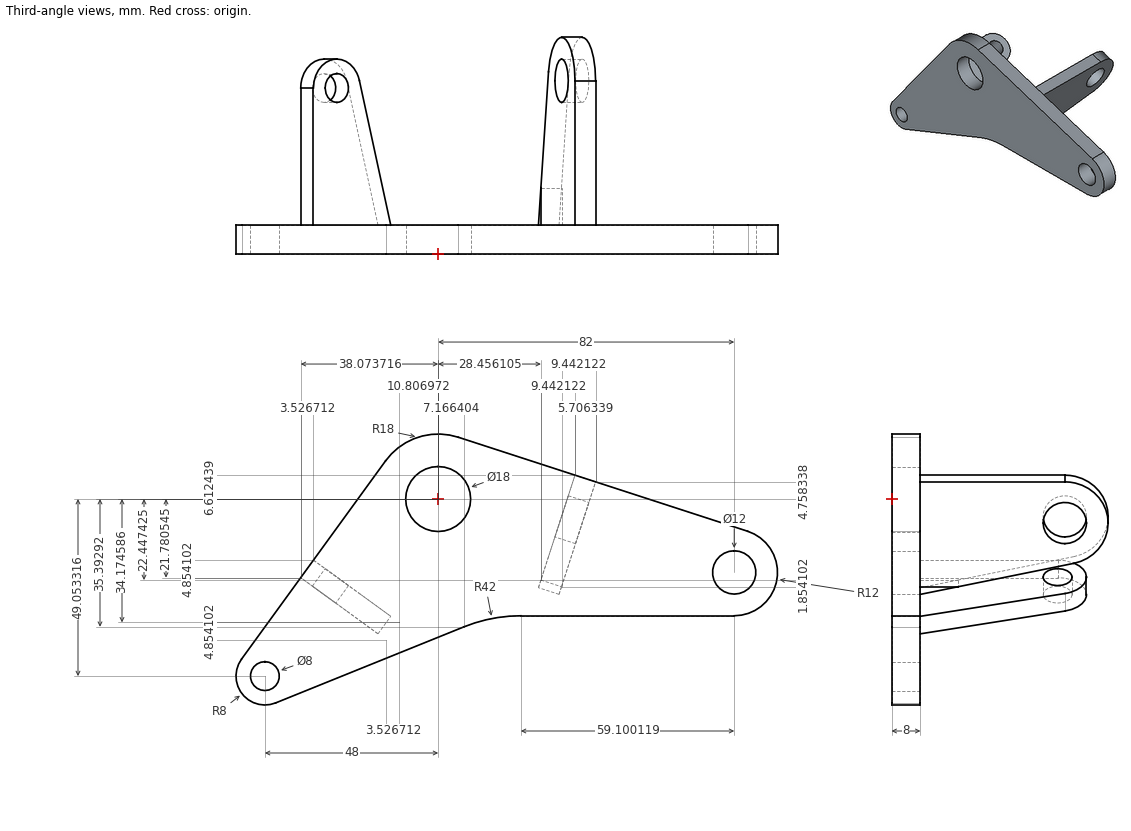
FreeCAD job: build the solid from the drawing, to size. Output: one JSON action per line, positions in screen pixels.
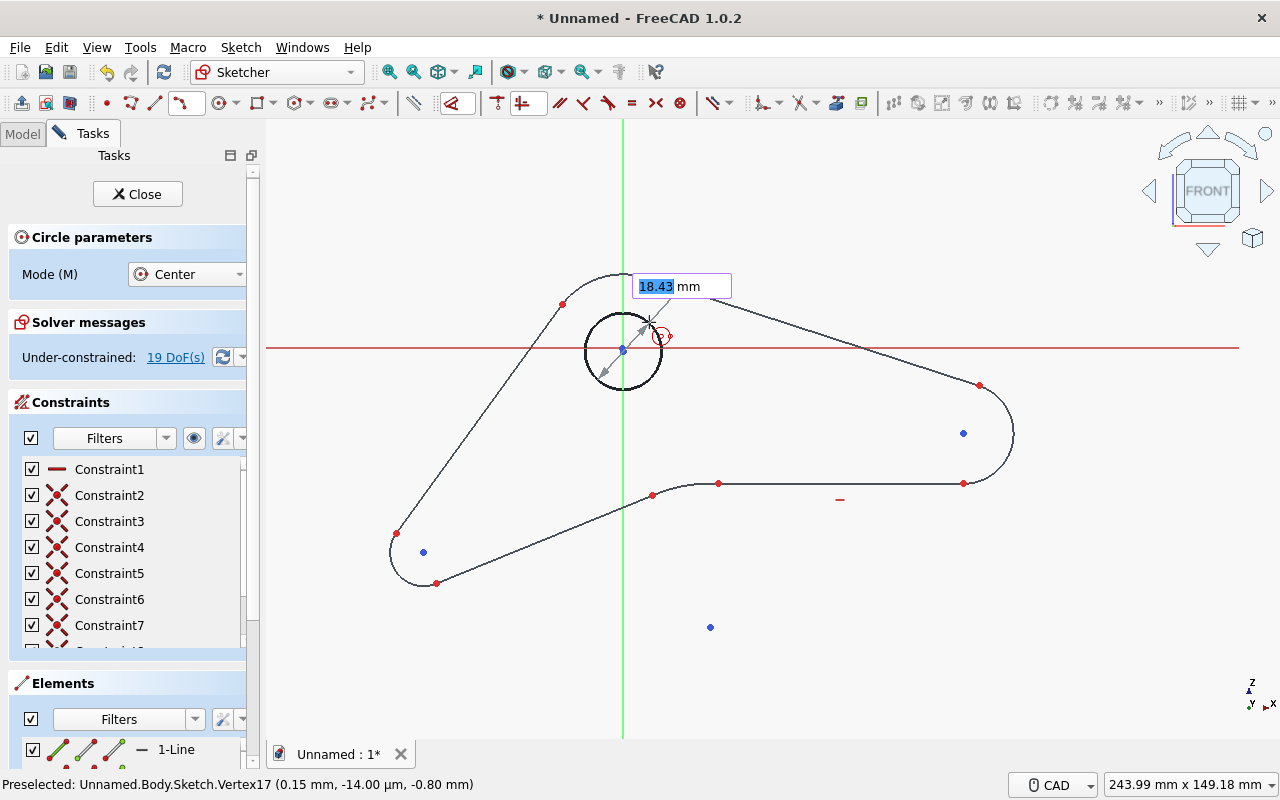
{"action": "type", "text": "18"}
{"action": "key", "text": "Return"}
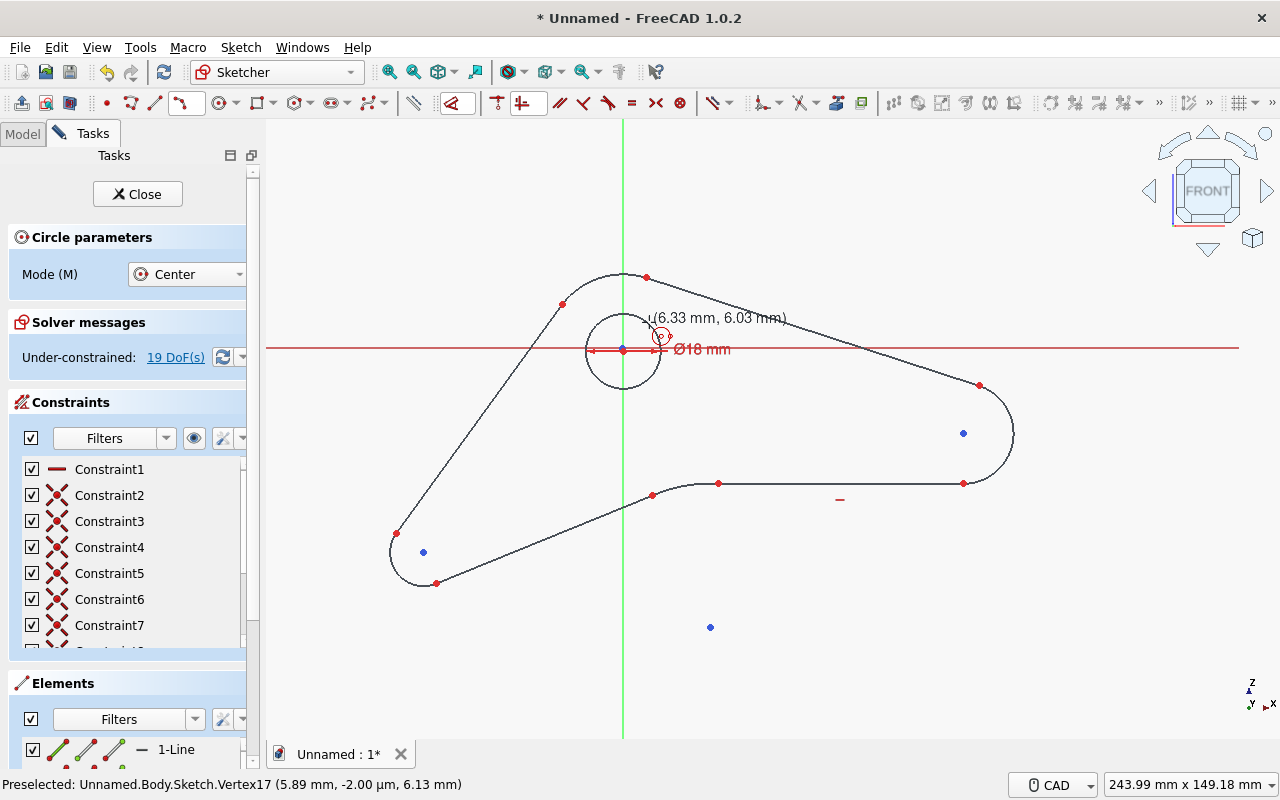
{"action": "left_click", "coordinate": [963, 433]}
{"action": "mouse_move", "coordinate": [981, 415]}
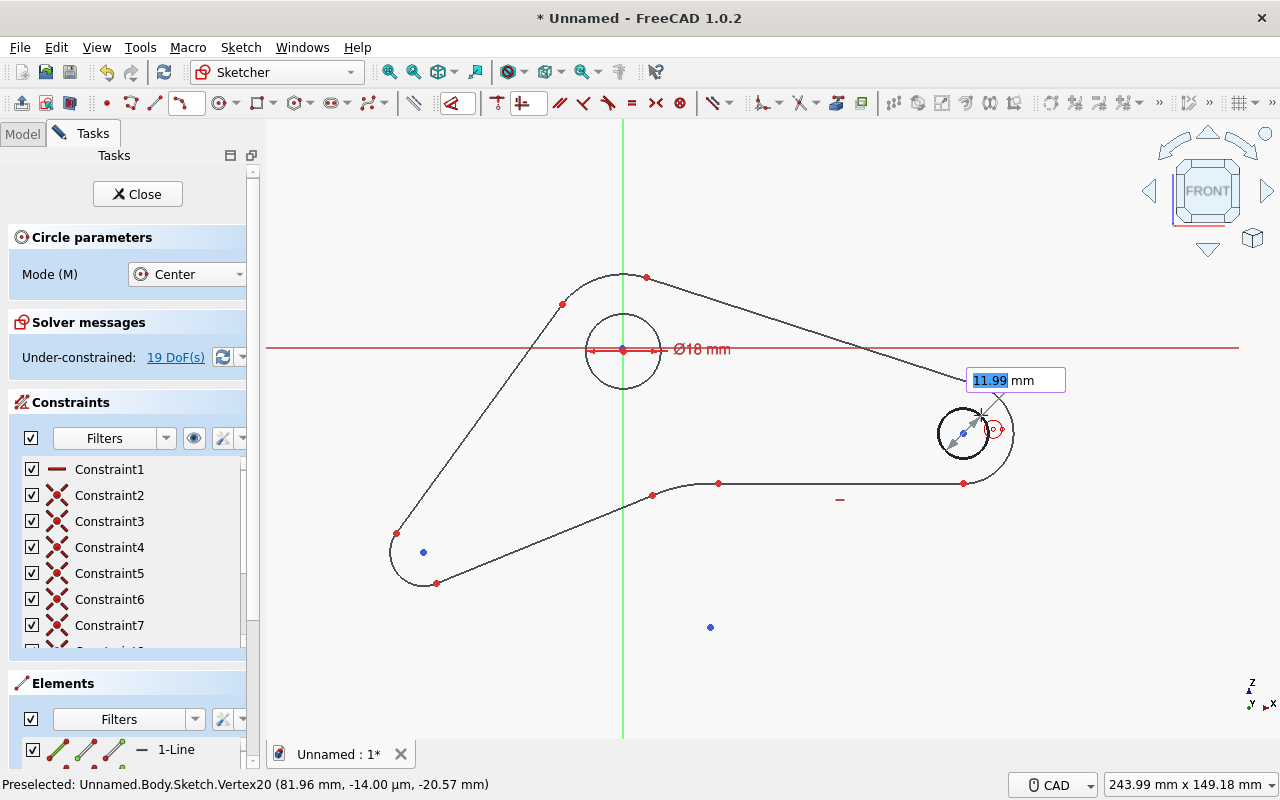
{"action": "type", "text": "12"}
{"action": "key", "text": "Return"}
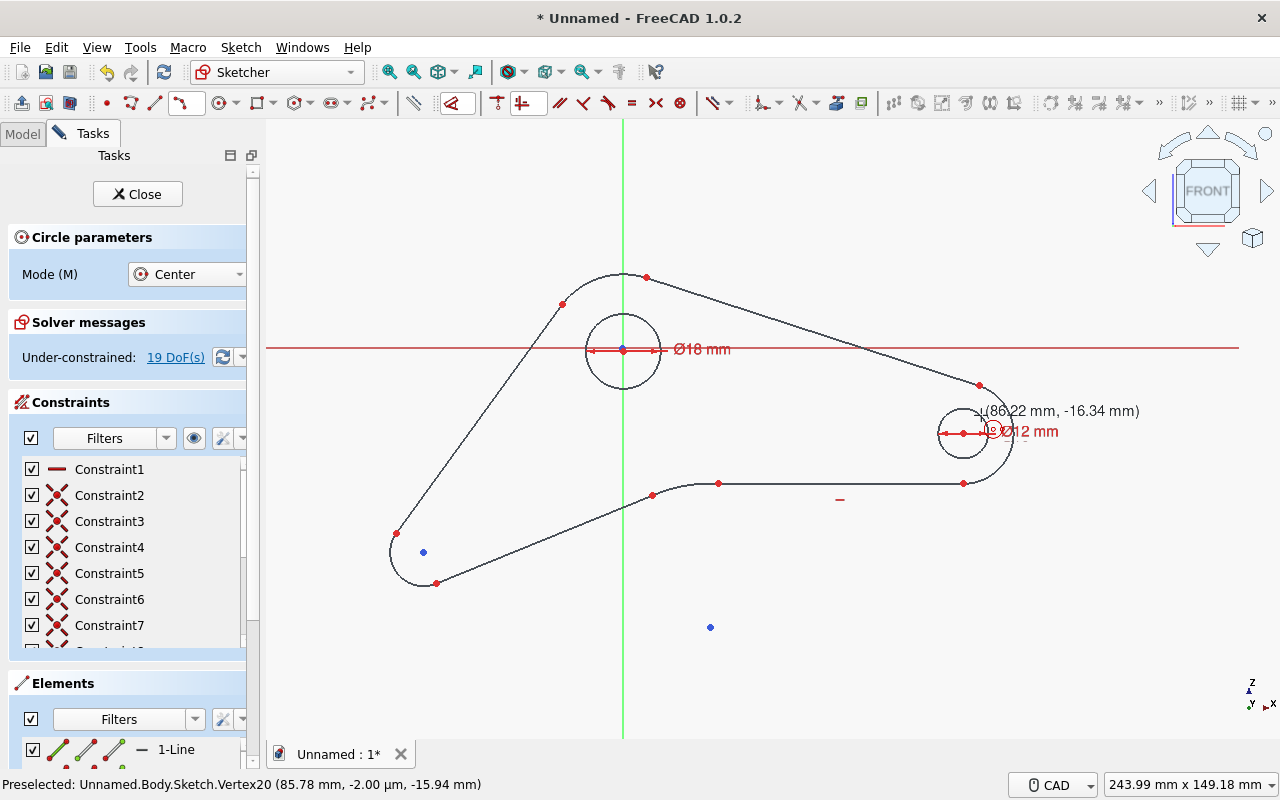
{"action": "scroll", "coordinate": [423, 552], "scroll_direction": "up", "scroll_amount": 2}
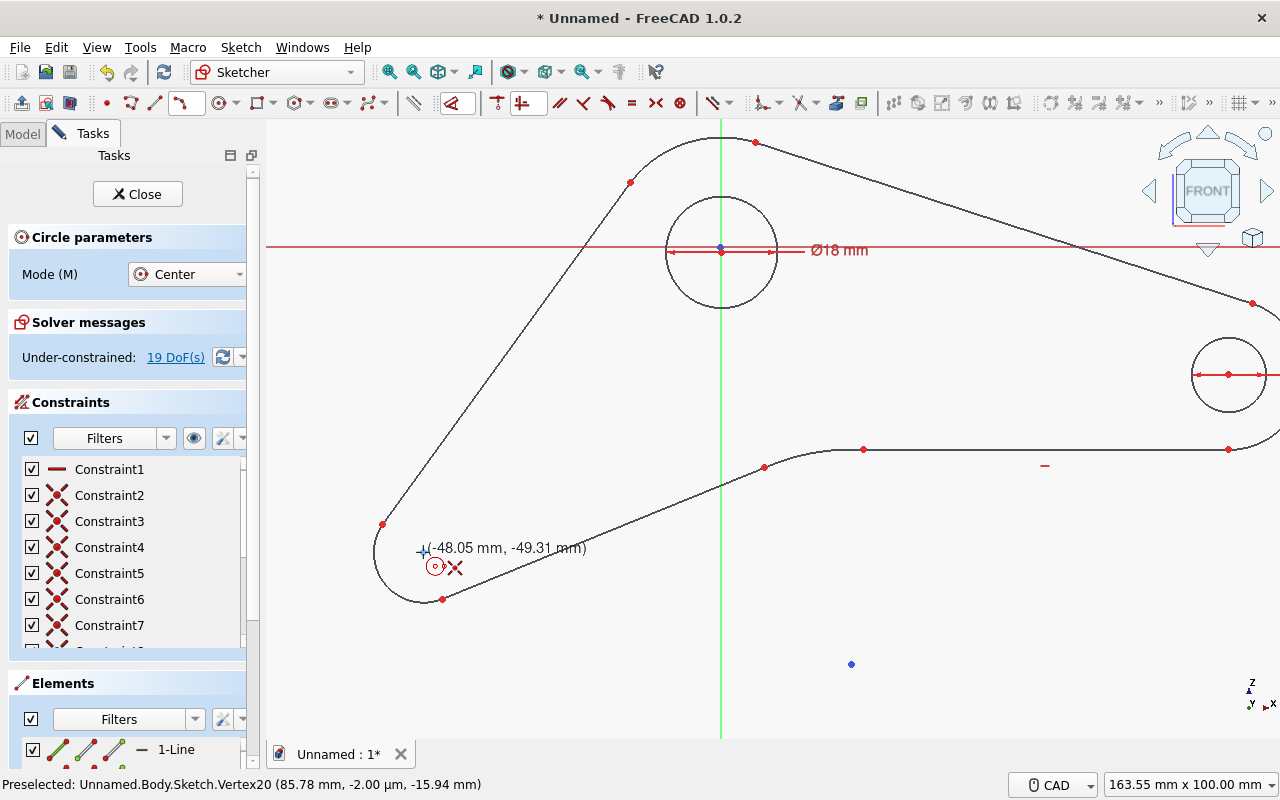
{"action": "left_click", "coordinate": [423, 552]}
{"action": "mouse_move", "coordinate": [441, 534]}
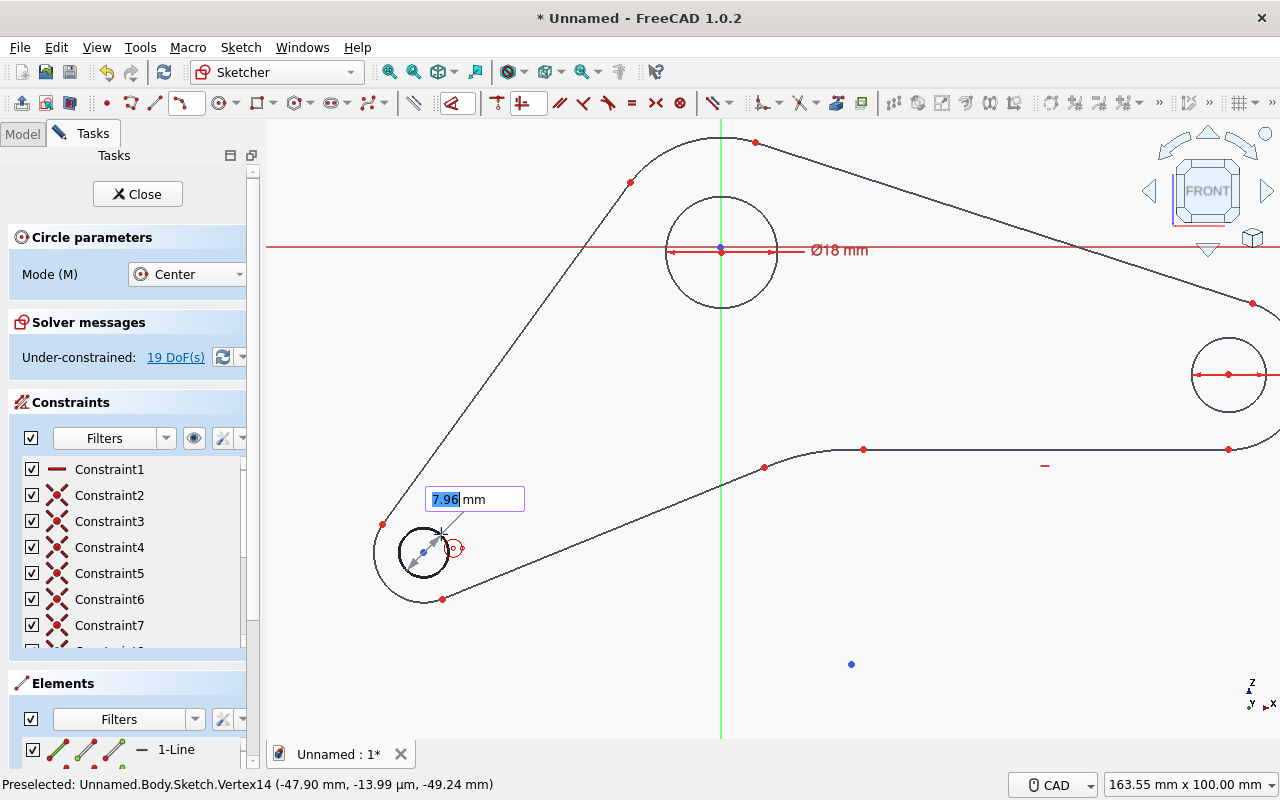
{"action": "type", "text": "8"}
{"action": "key", "text": "Return"}
{"action": "key", "text": "Escape"}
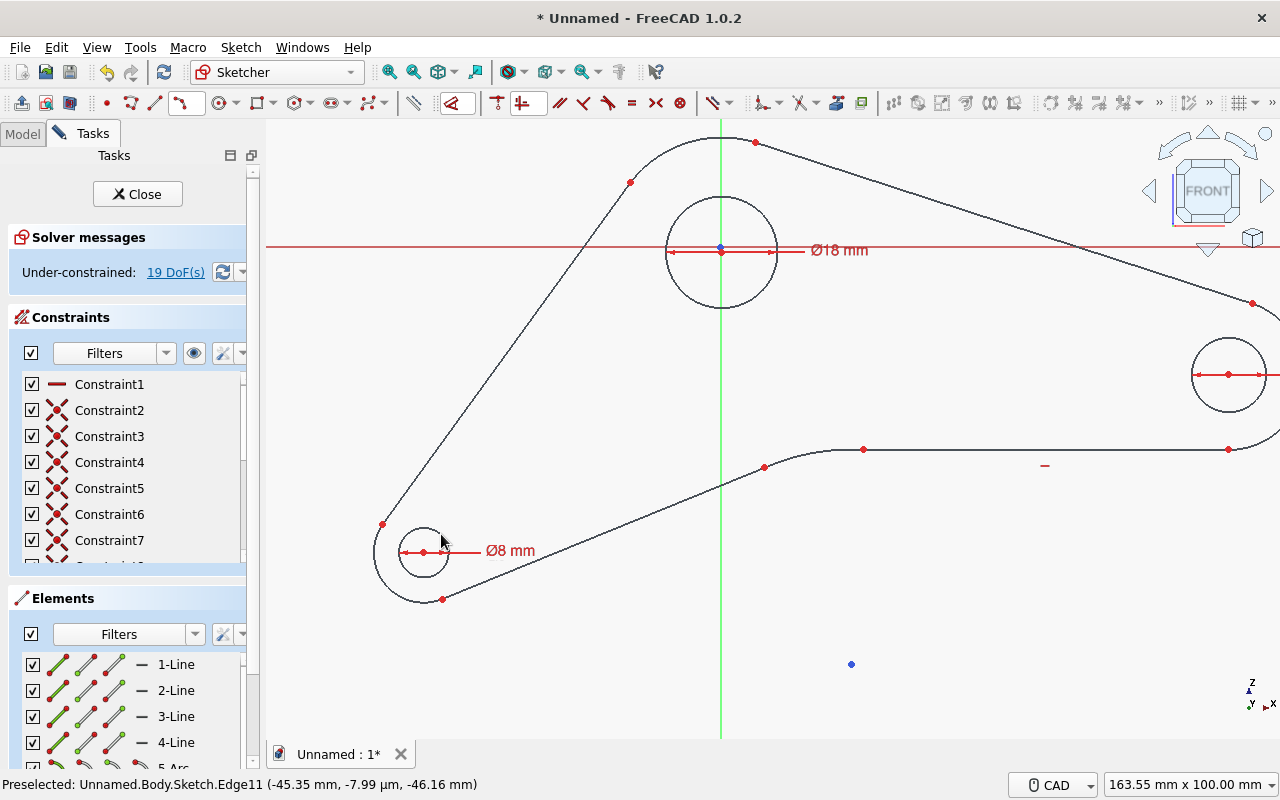
{"action": "left_click", "coordinate": [973, 450]}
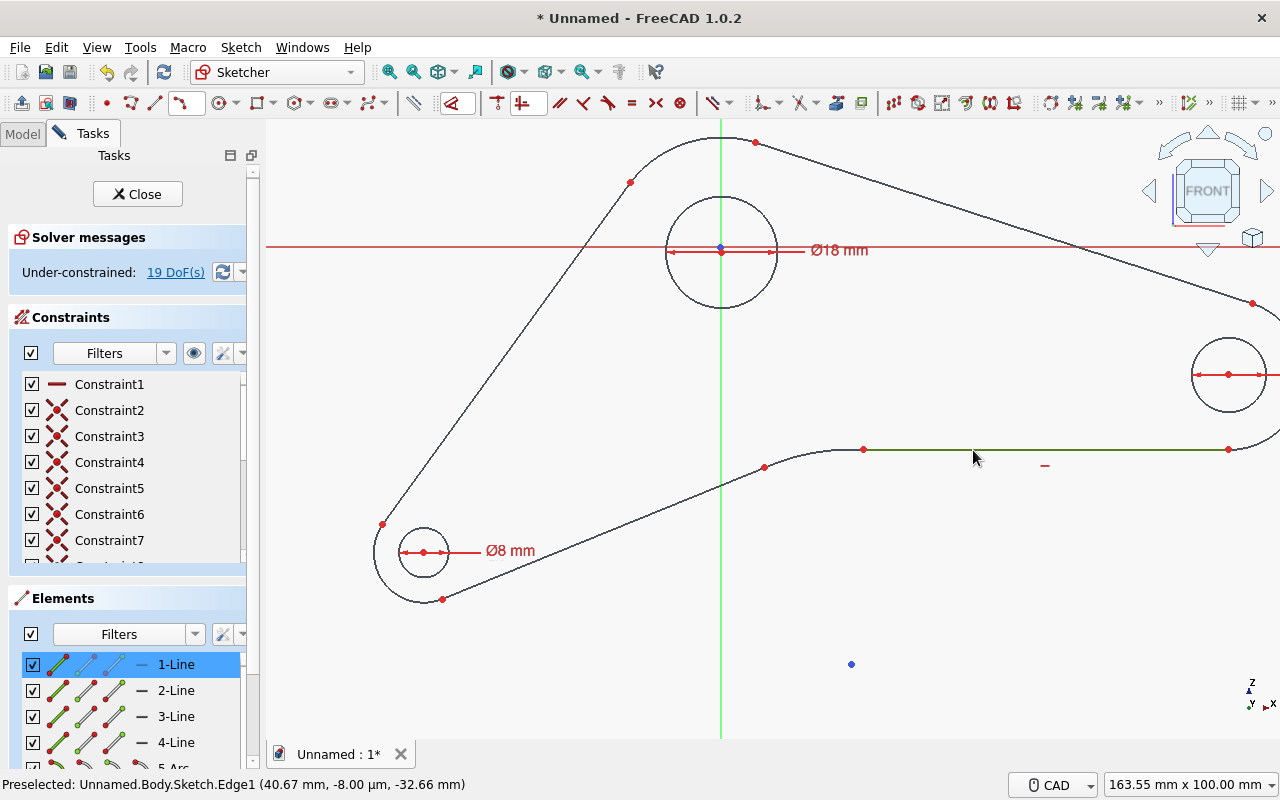
{"action": "scroll", "coordinate": [423, 550], "scroll_direction": "down", "scroll_amount": 2}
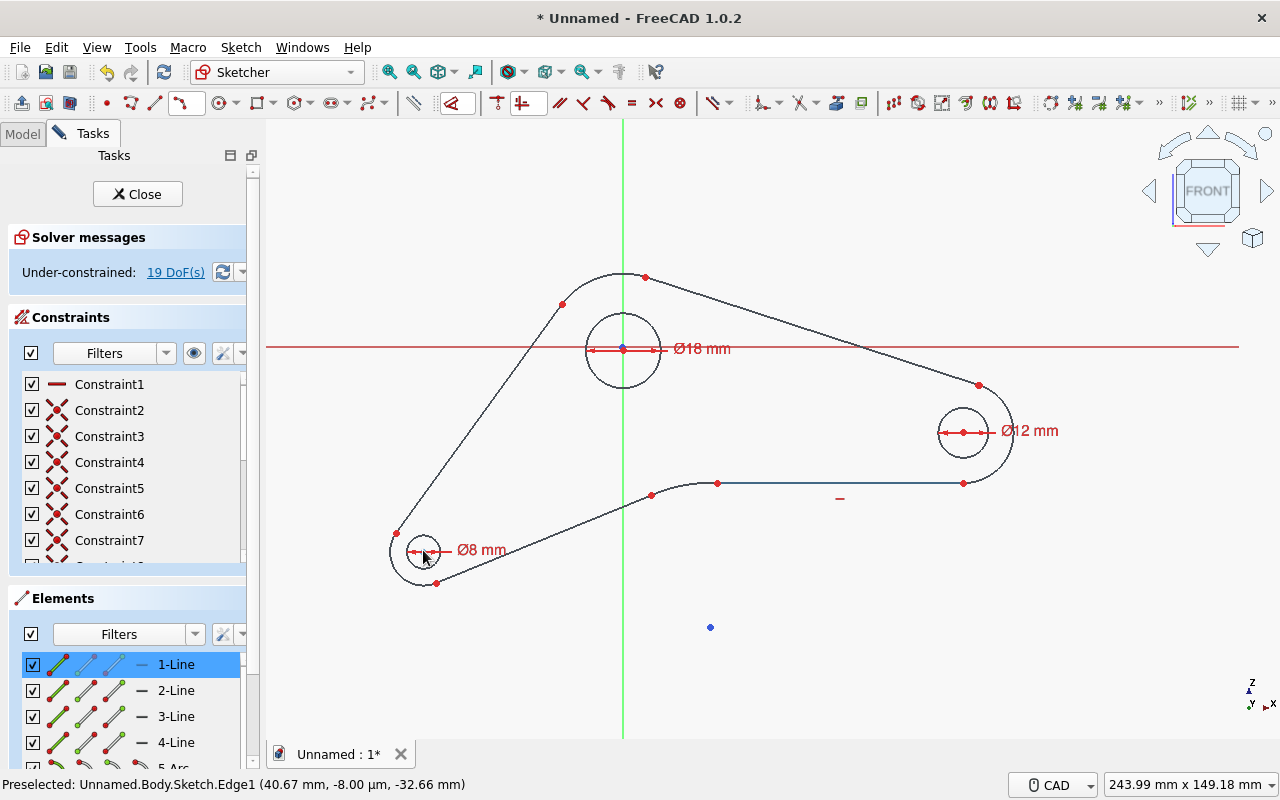
{"action": "left_click", "coordinate": [1001, 466]}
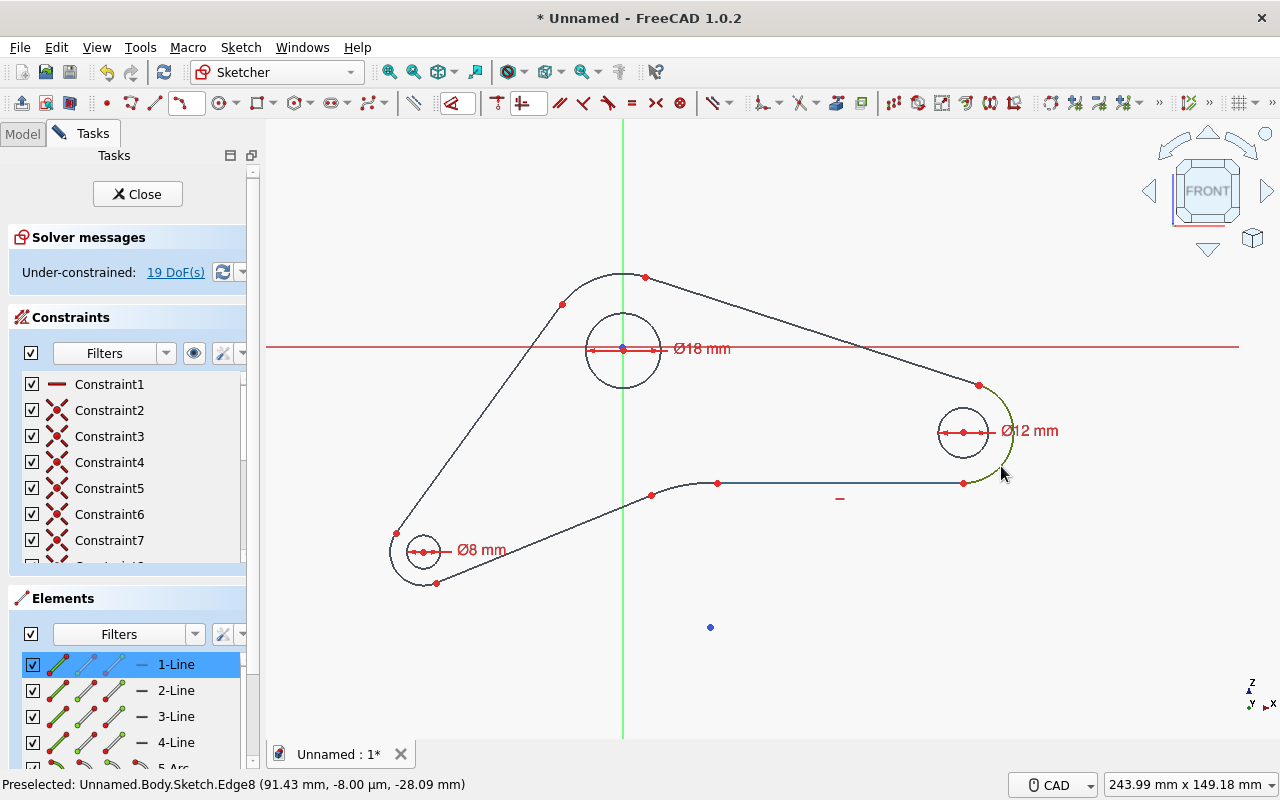
{"action": "left_click", "coordinate": [608, 104]}